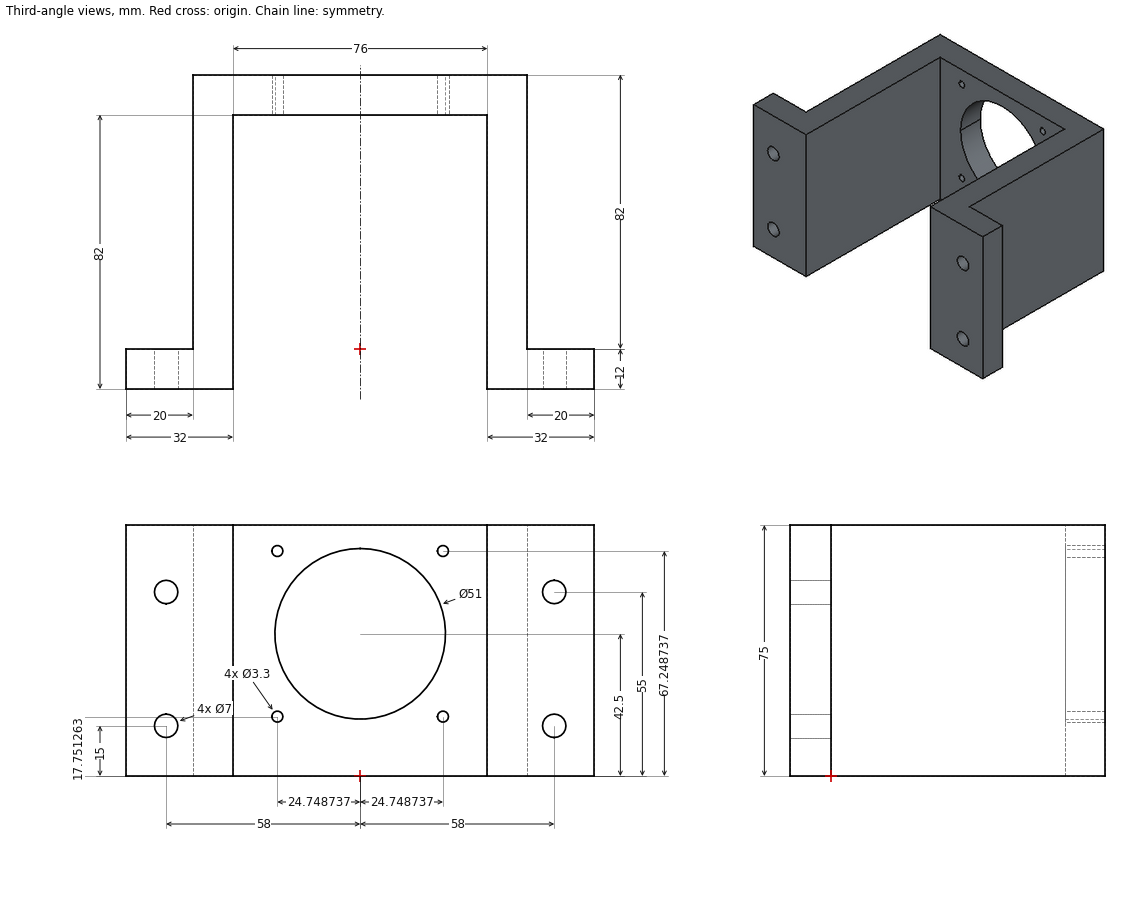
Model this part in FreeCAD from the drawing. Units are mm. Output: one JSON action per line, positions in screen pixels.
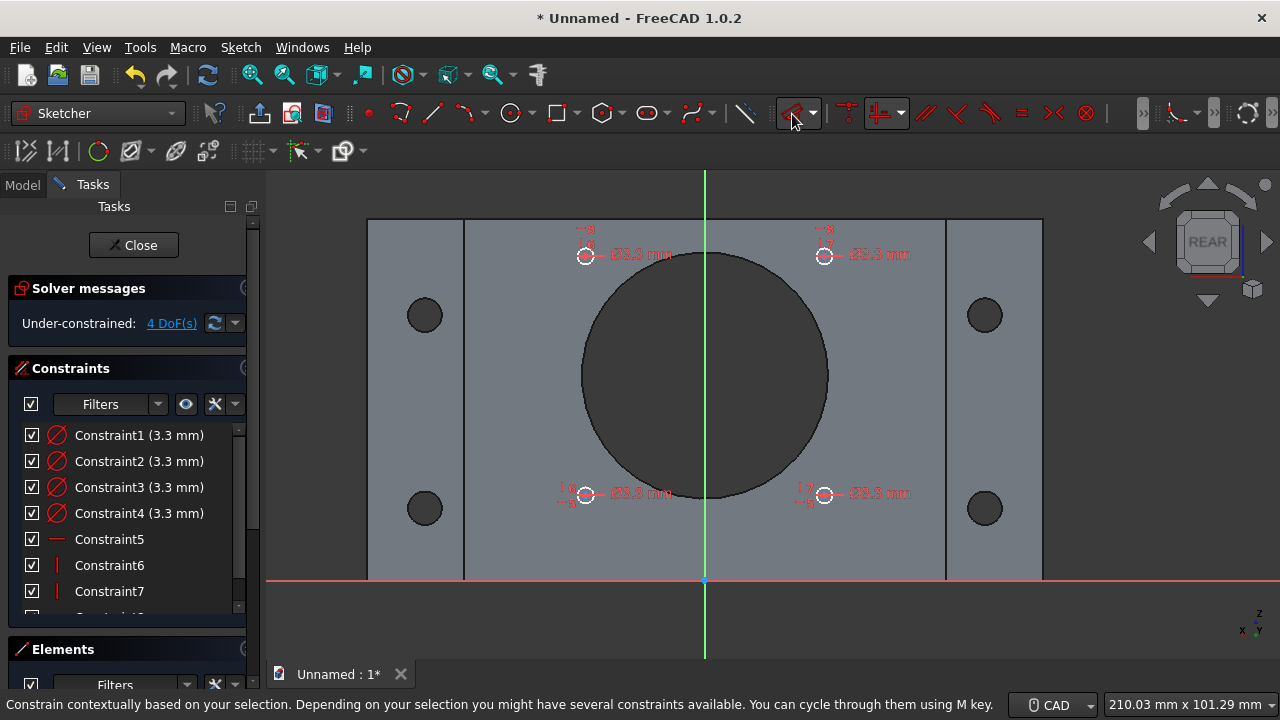
{"action": "left_click", "coordinate": [824, 495]}
{"action": "left_click", "coordinate": [765, 615]}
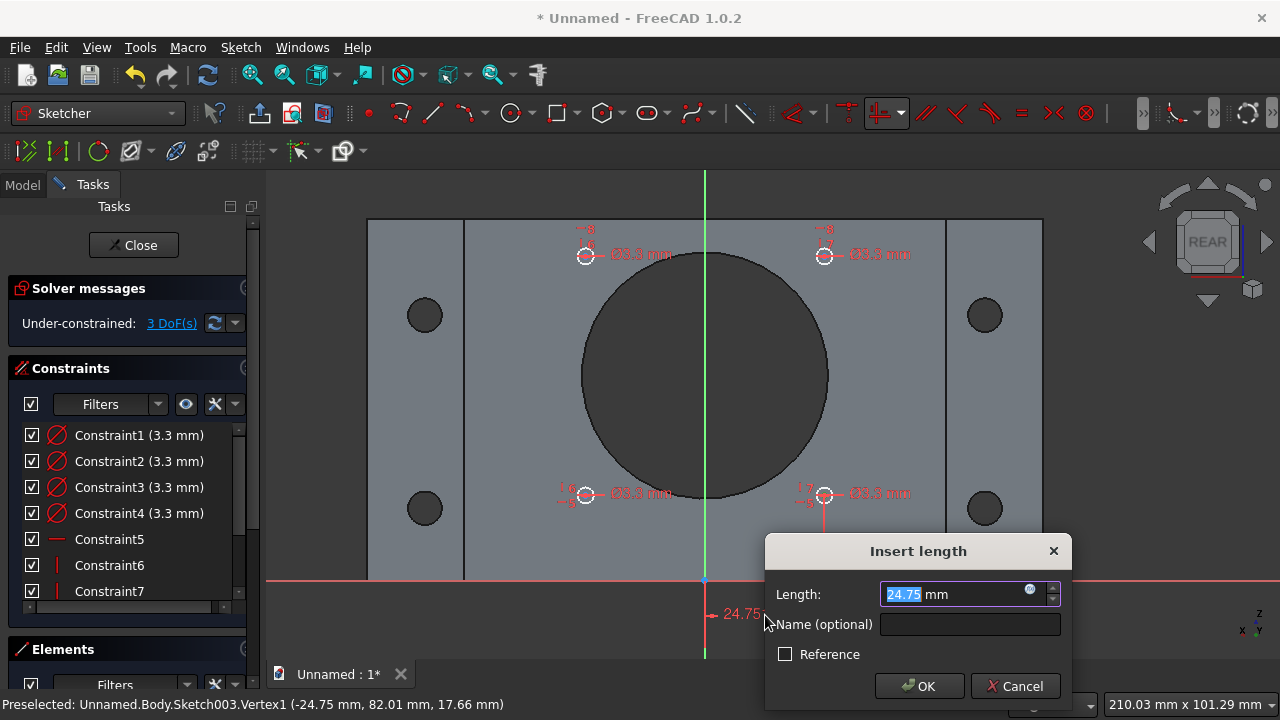
{"action": "type", "text": "24.748737"}
{"action": "key", "text": "Return"}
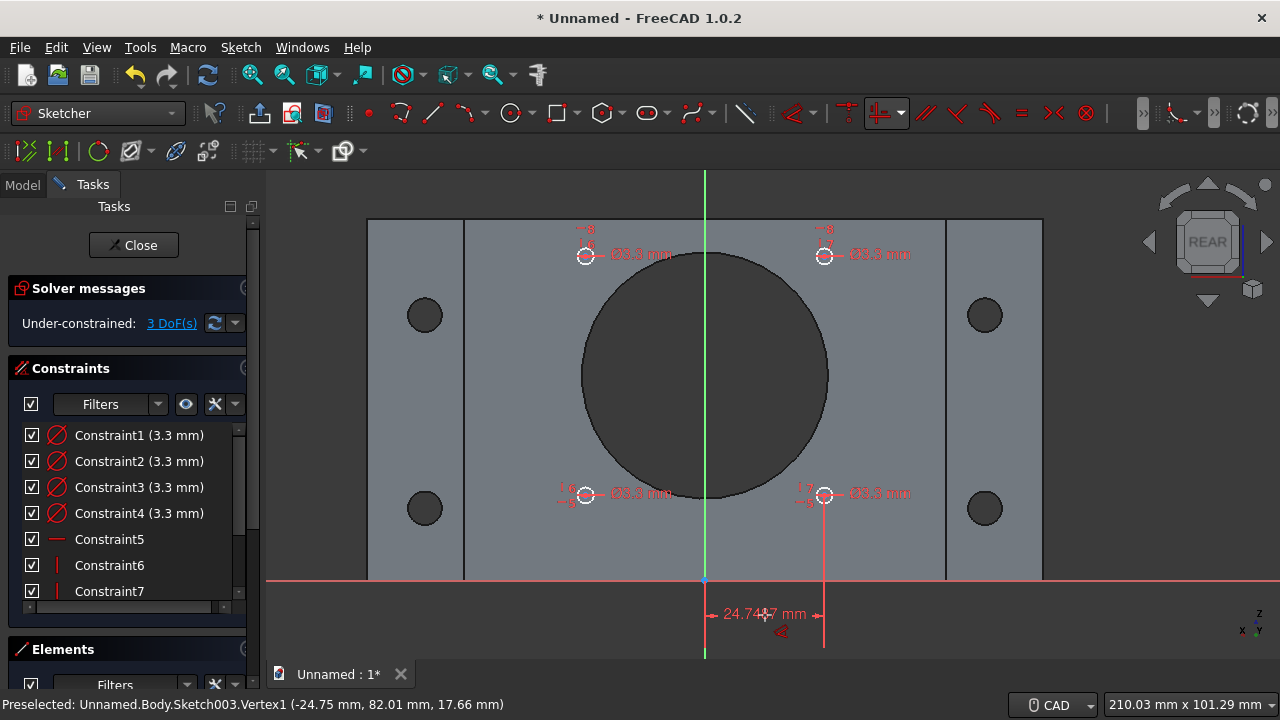
{"action": "left_click", "coordinate": [824, 495]}
{"action": "left_click", "coordinate": [858, 538]}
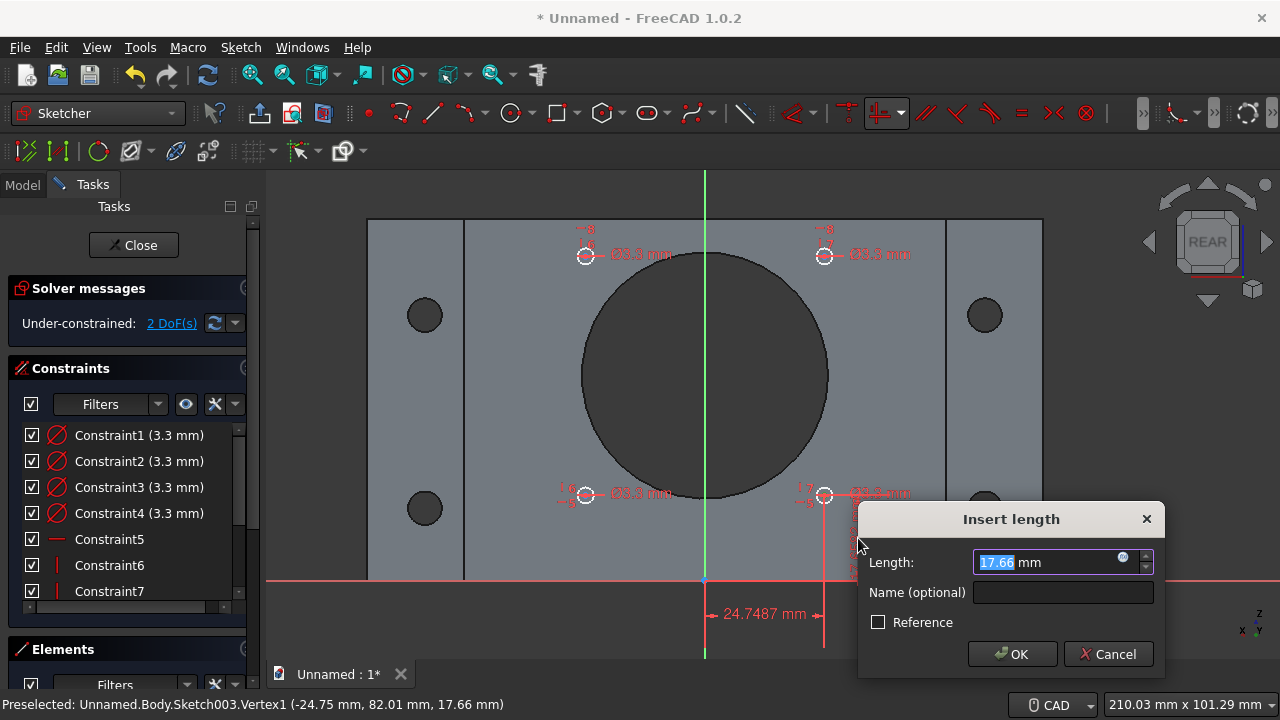
{"action": "type", "text": "17.751263"}
{"action": "key", "text": "Return"}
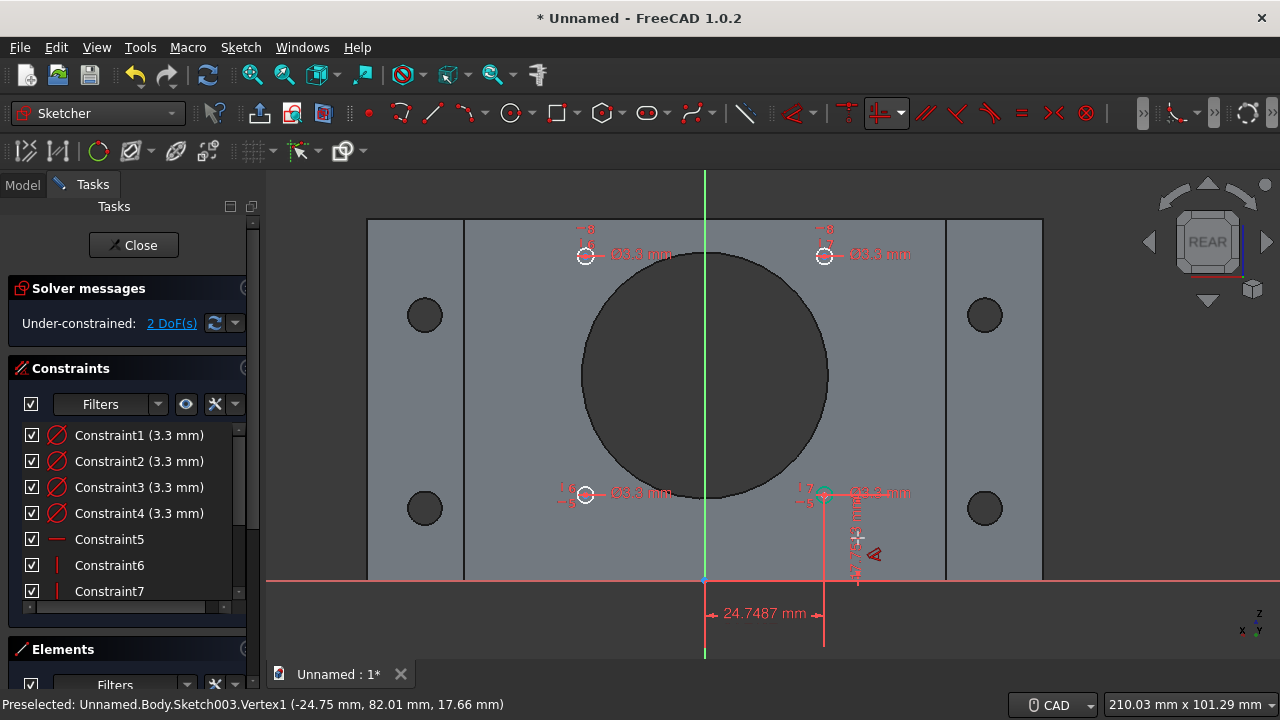
{"action": "left_click", "coordinate": [586, 495]}
{"action": "left_click", "coordinate": [645, 615]}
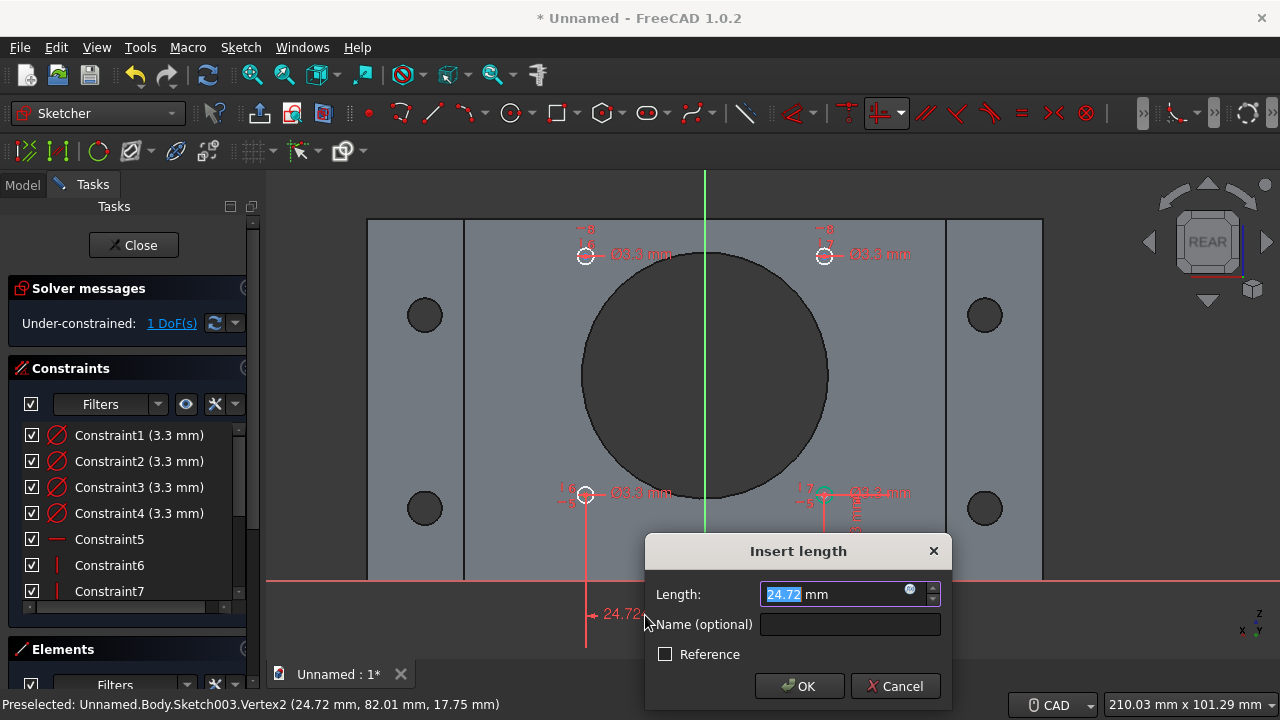
{"action": "type", "text": "24.748737"}
{"action": "key", "text": "Return"}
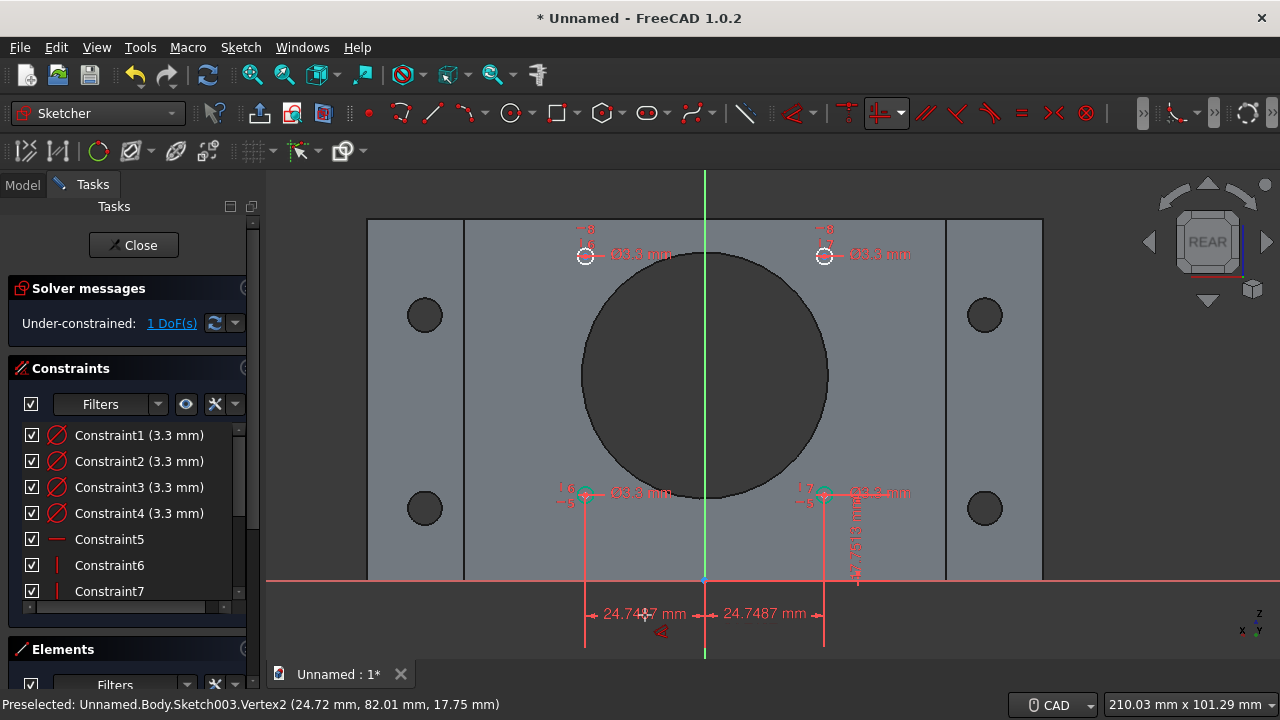
{"action": "left_click", "coordinate": [586, 256]}
{"action": "left_click", "coordinate": [552, 419]}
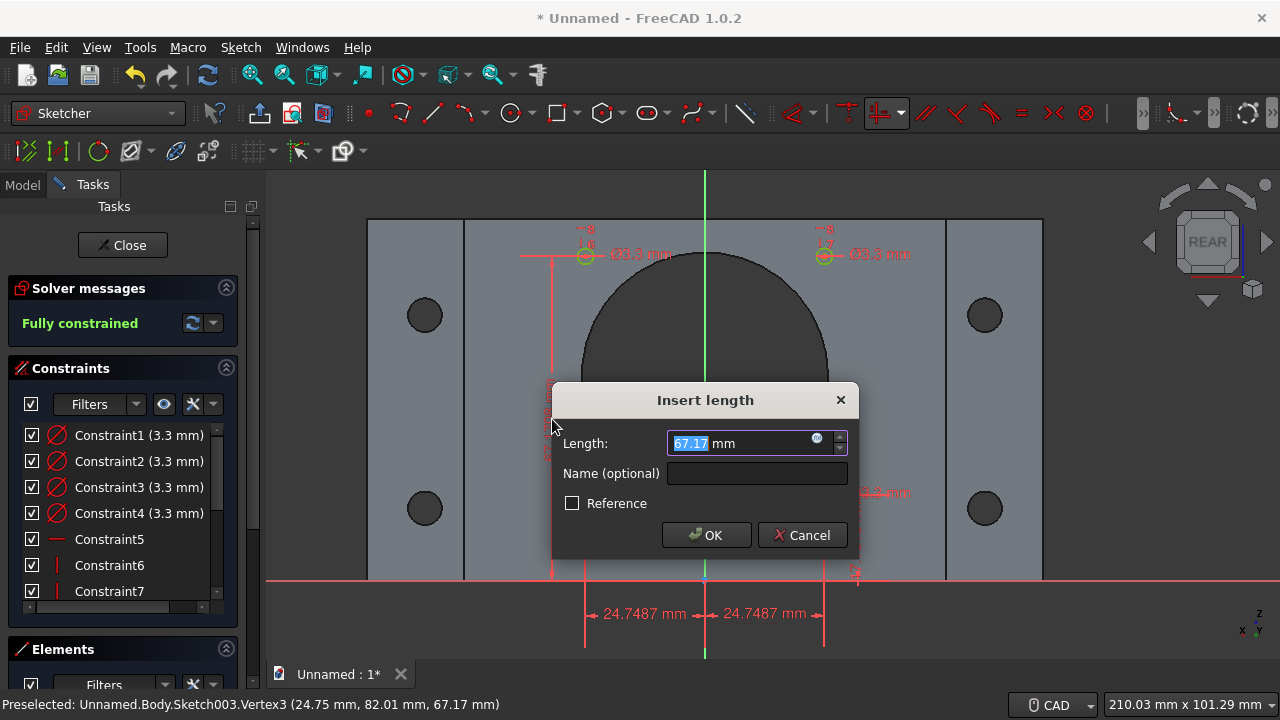
{"action": "type", "text": "67.248737"}
{"action": "key", "text": "Return"}
{"action": "key", "text": "Escape"}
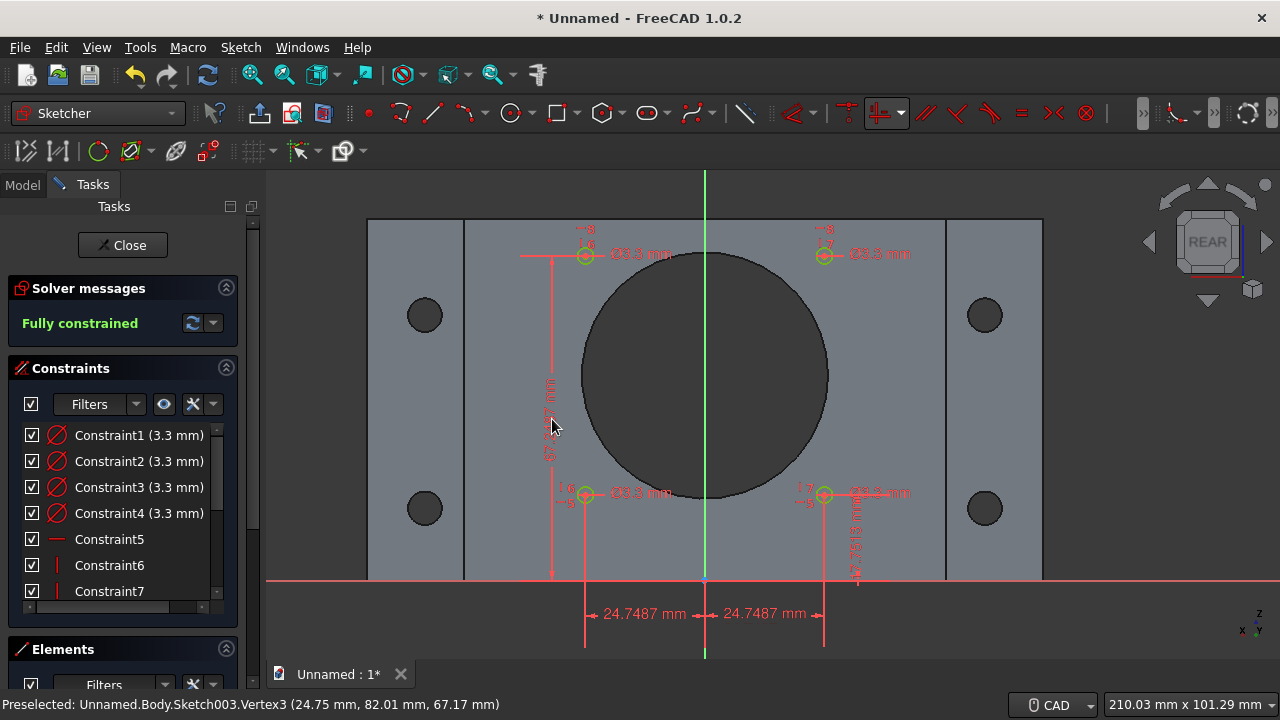
{"action": "left_click", "coordinate": [123, 245]}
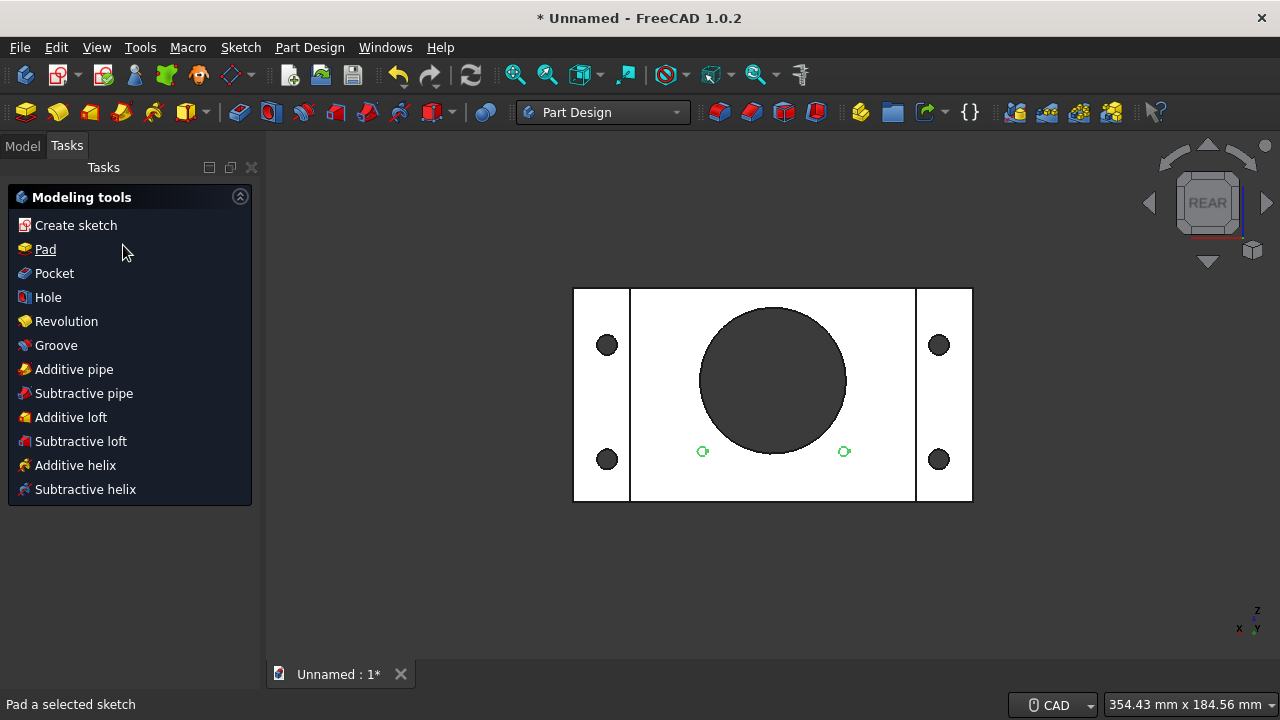
{"action": "left_click", "coordinate": [240, 112]}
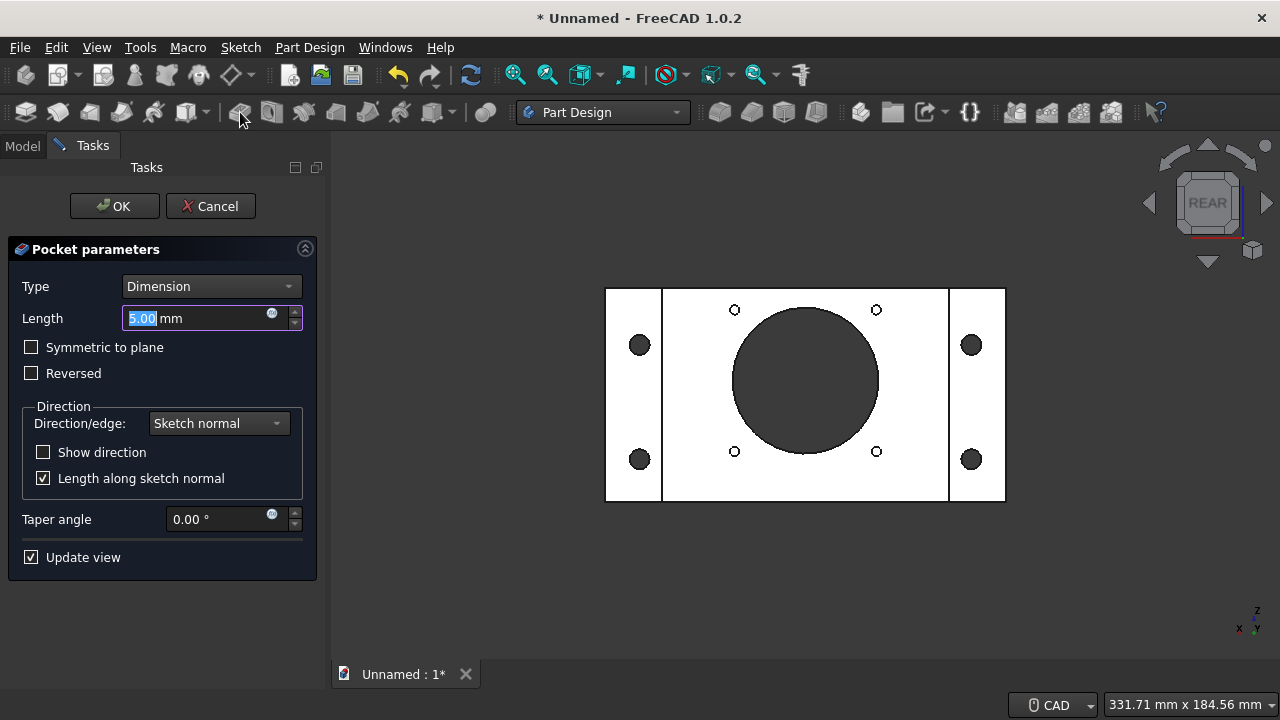
{"action": "left_click", "coordinate": [212, 286]}